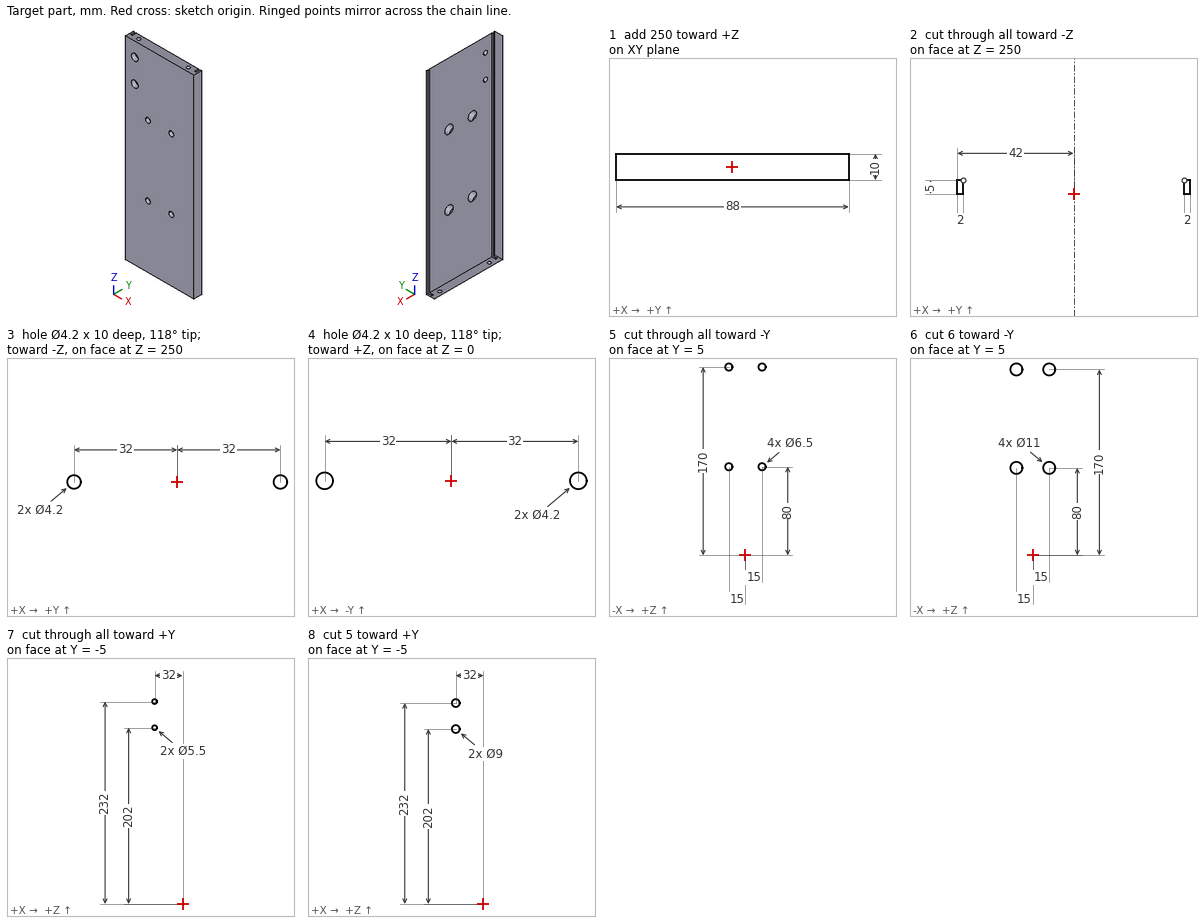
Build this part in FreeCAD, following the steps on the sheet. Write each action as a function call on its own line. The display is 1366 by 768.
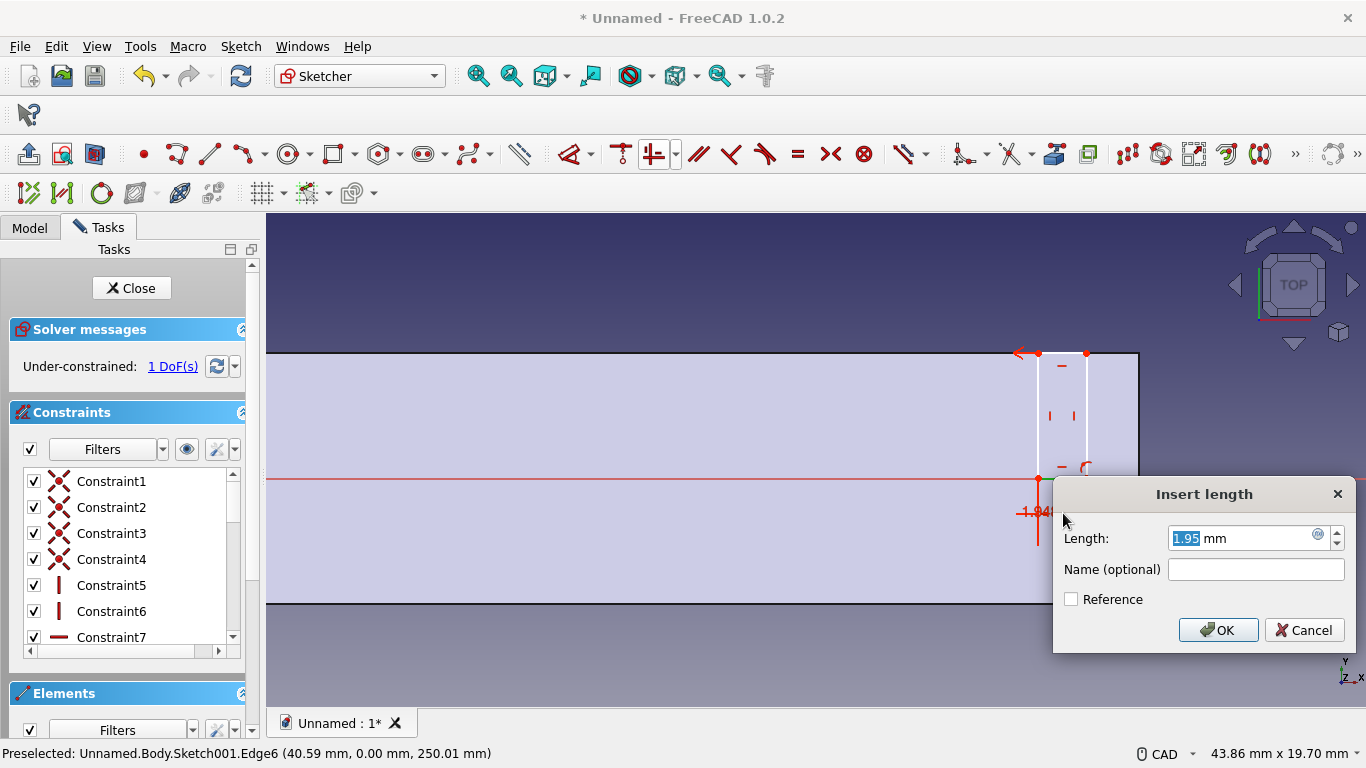
text(2)
key(Return)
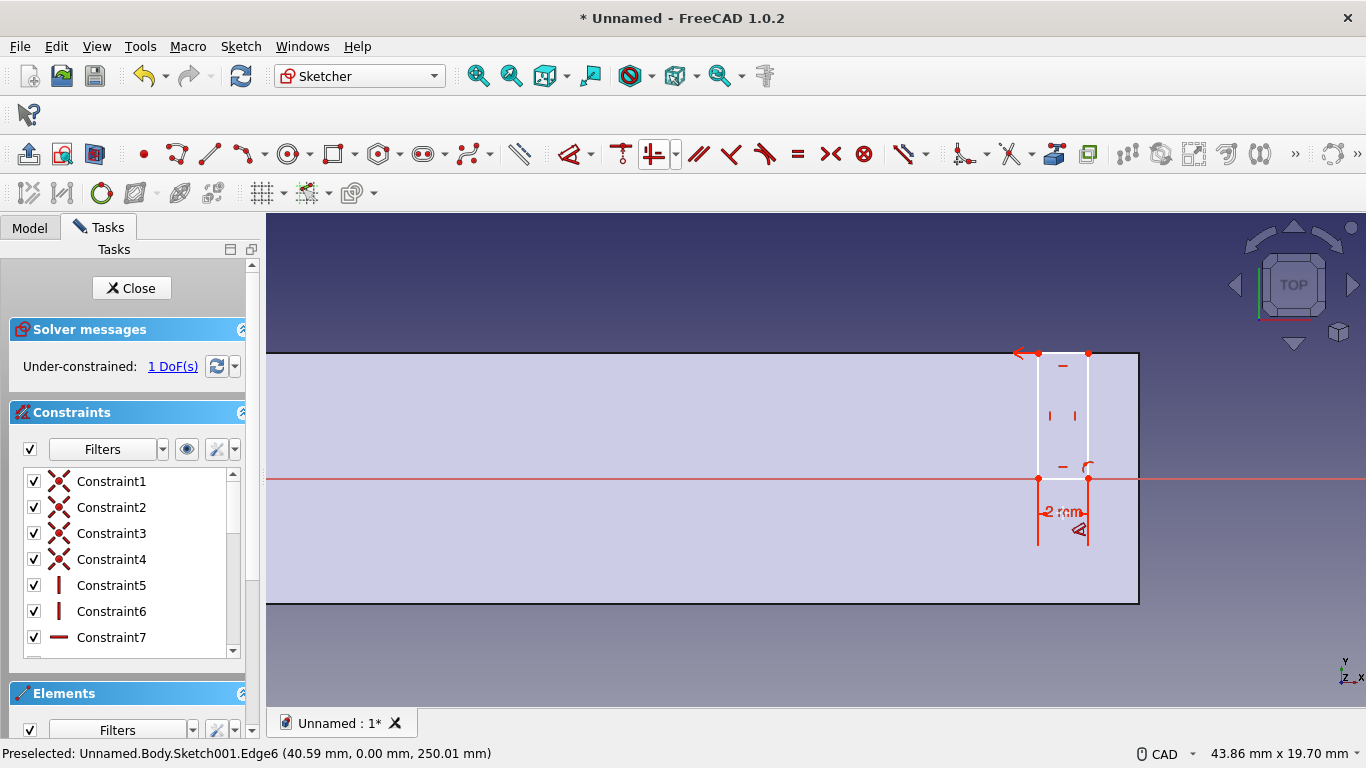
scroll(1055, 479, down, 6)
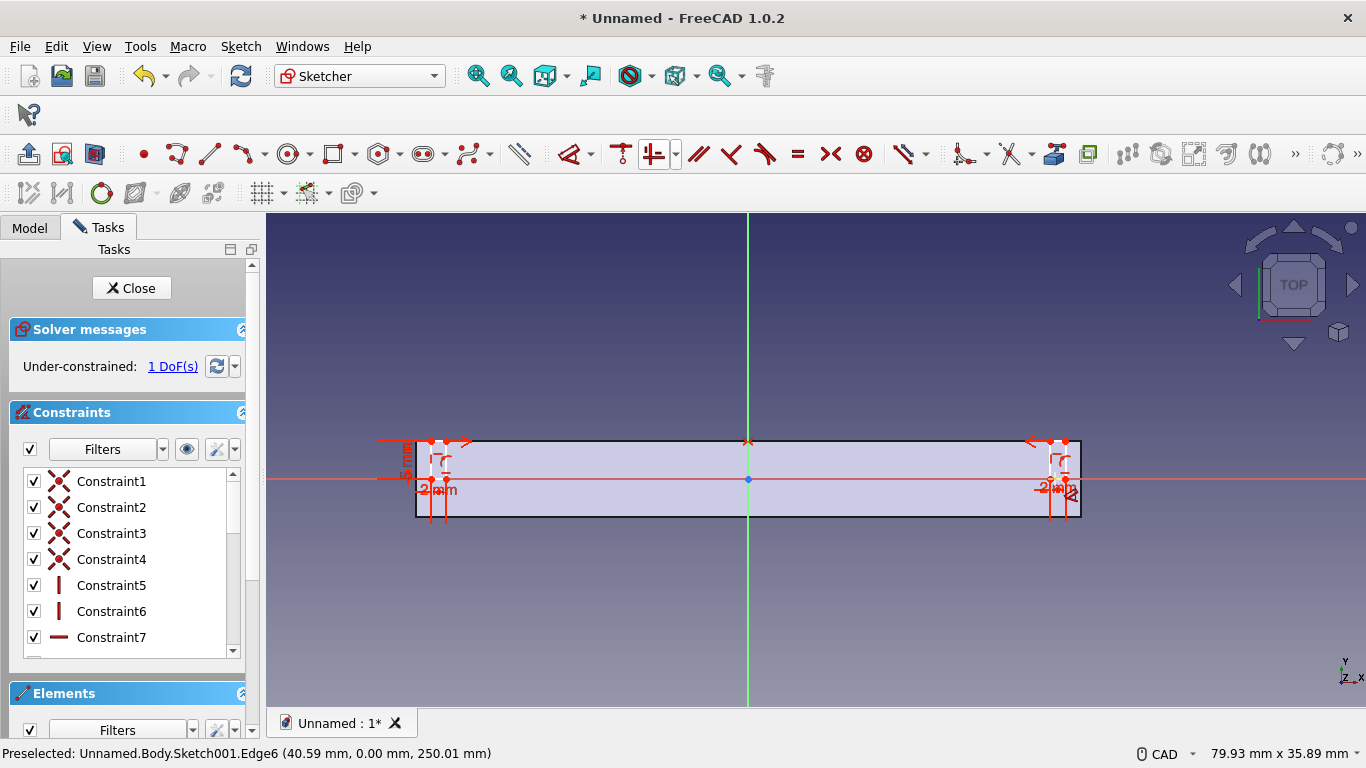
click(431, 441)
click(590, 513)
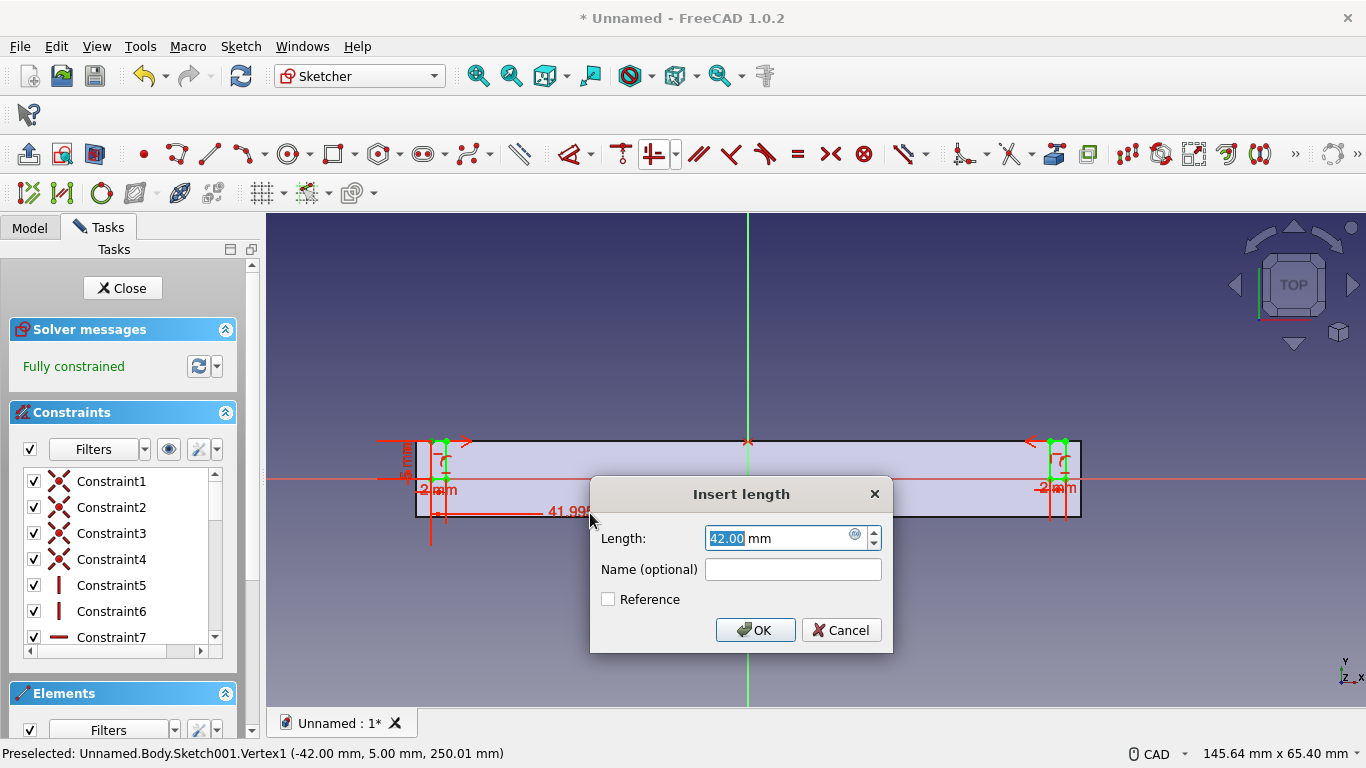
text(42)
key(Return)
key(Escape)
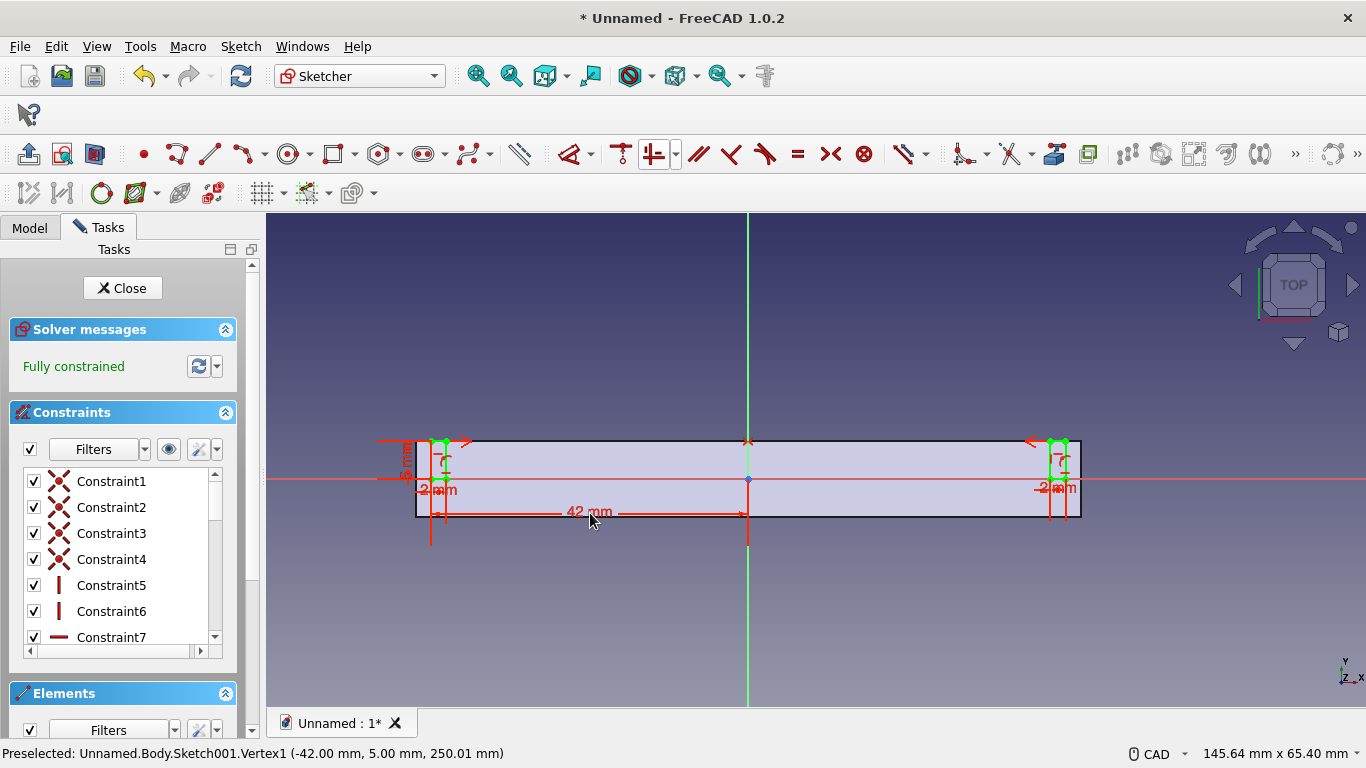
click(123, 288)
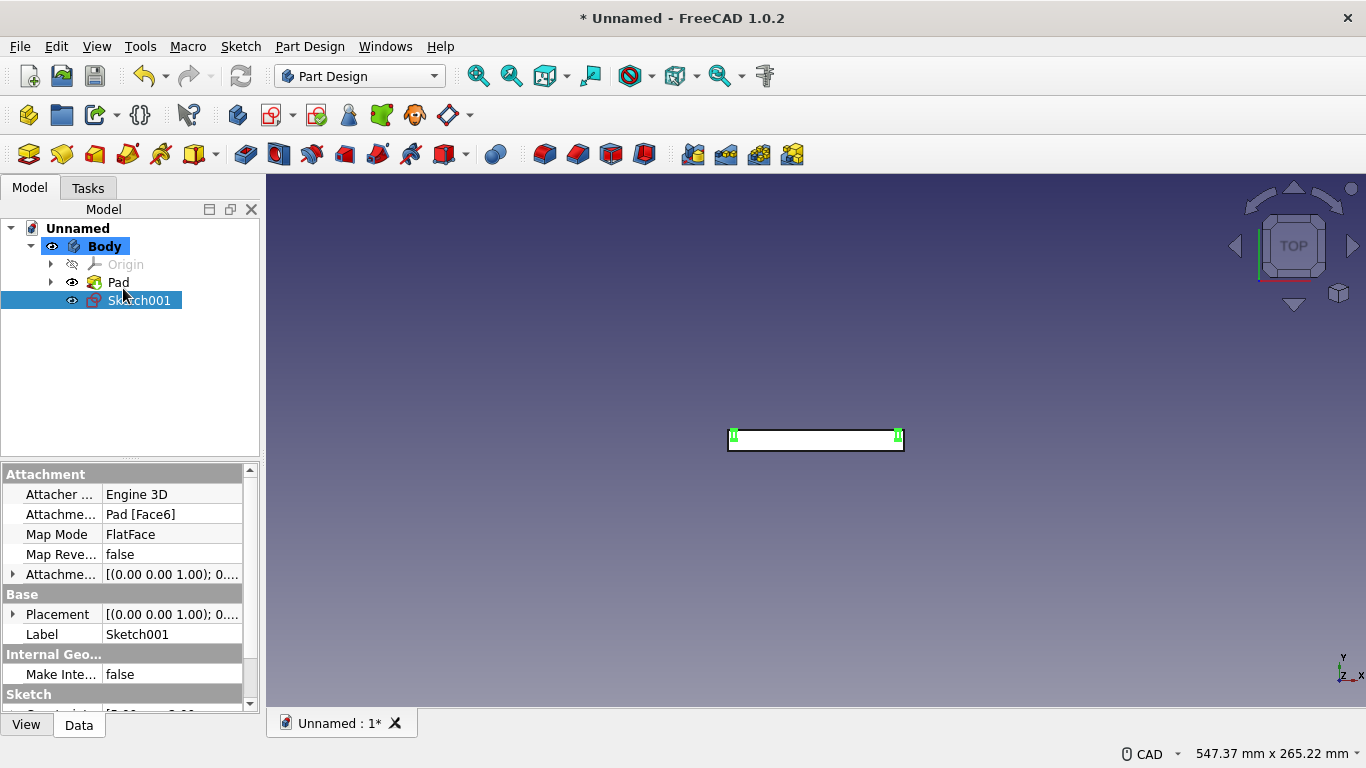
click(246, 154)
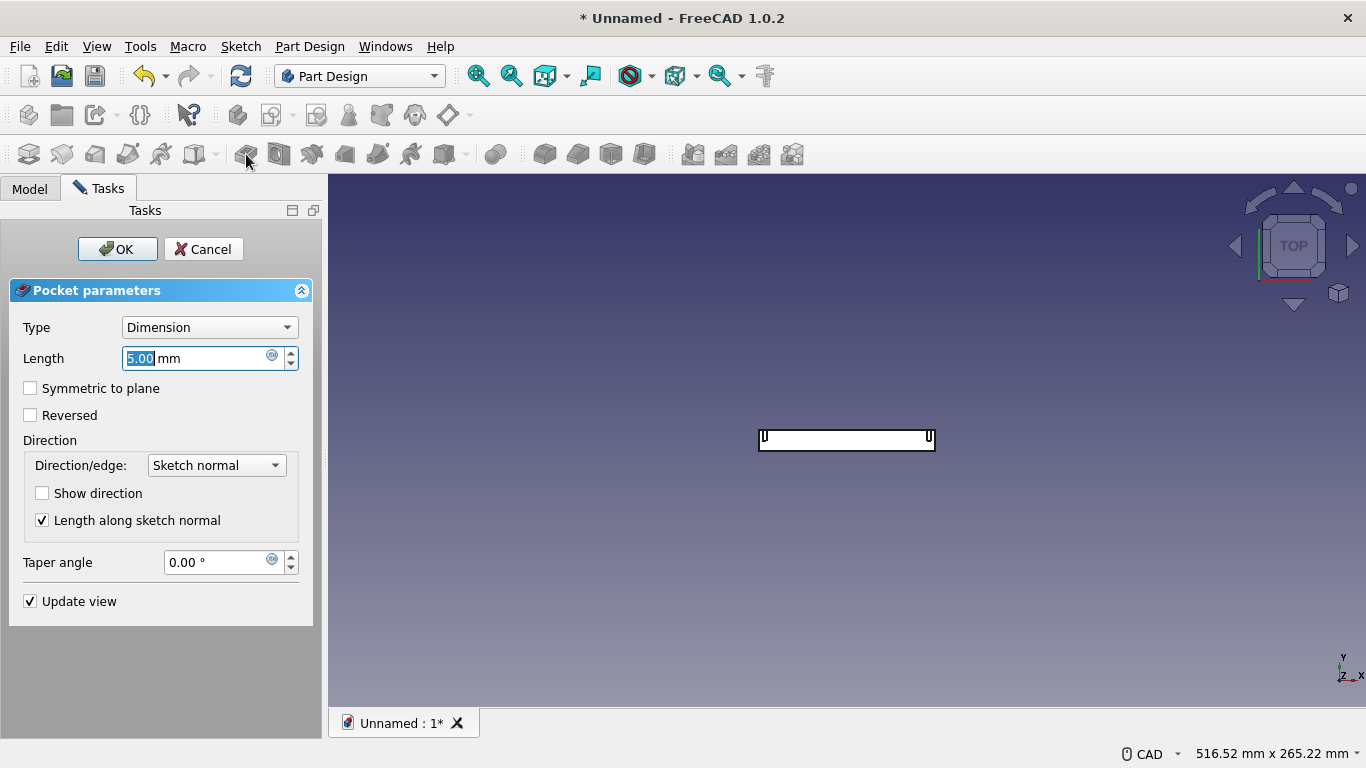
click(210, 328)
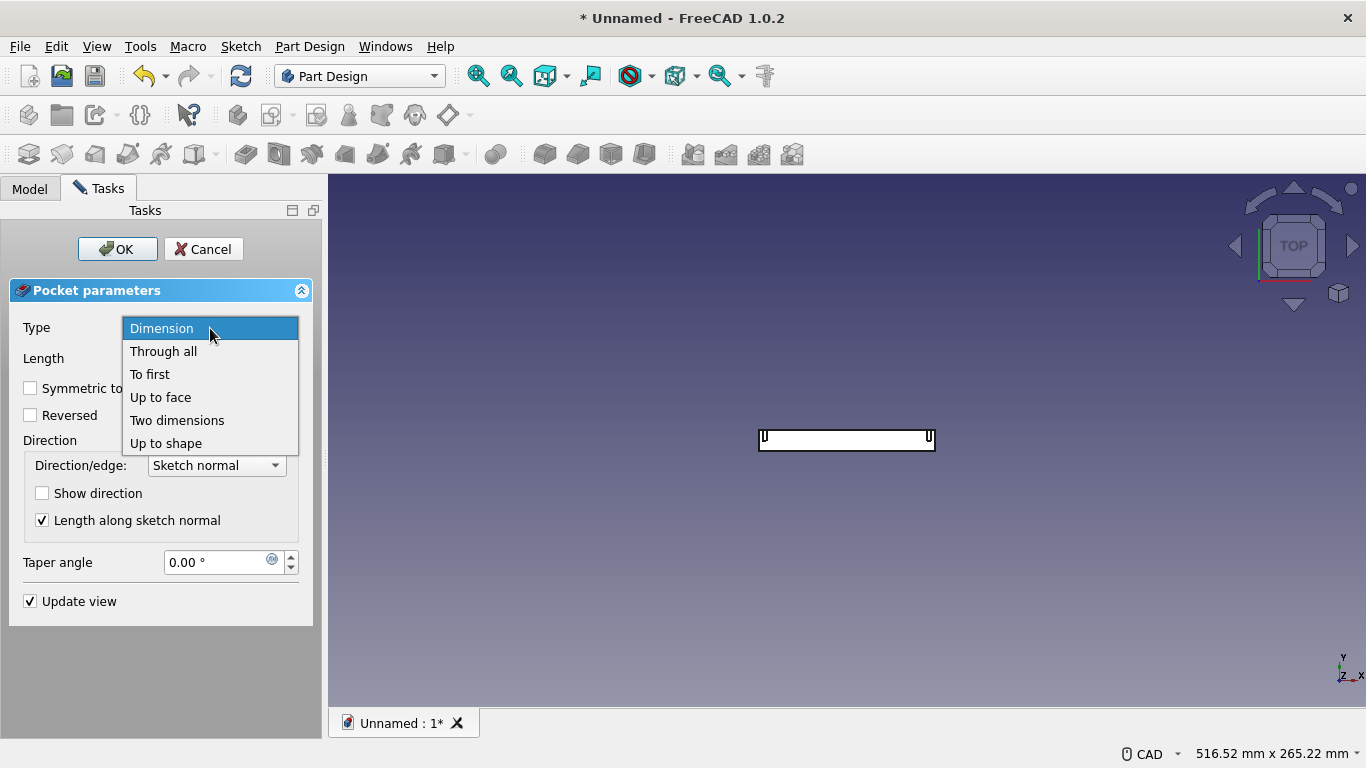
click(208, 352)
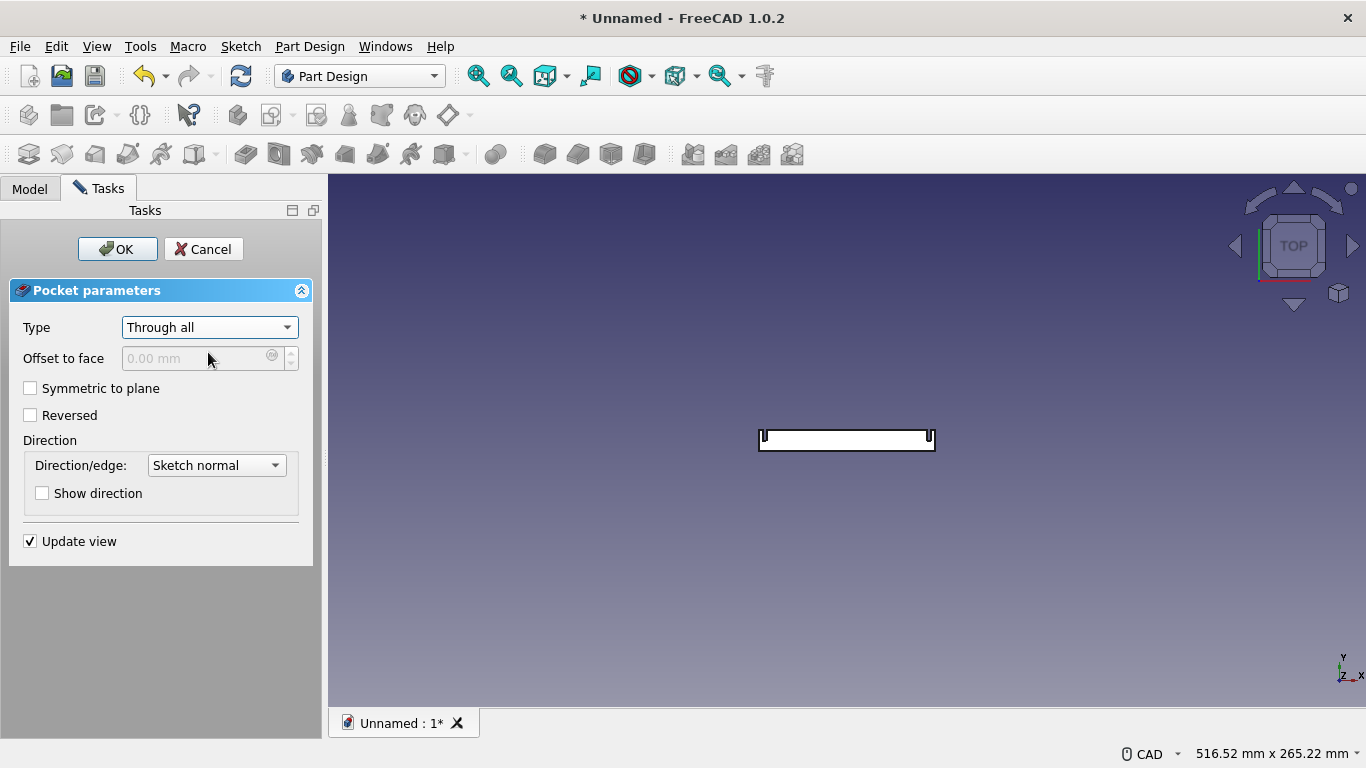
click(118, 249)